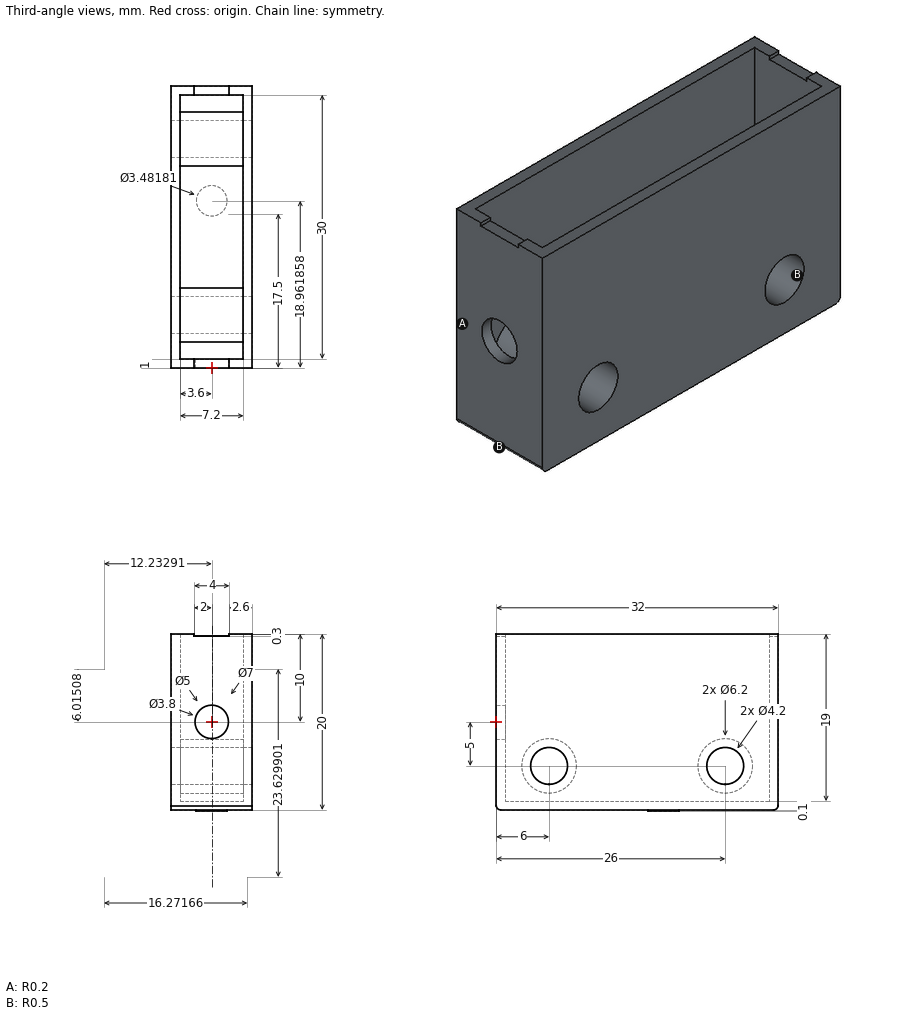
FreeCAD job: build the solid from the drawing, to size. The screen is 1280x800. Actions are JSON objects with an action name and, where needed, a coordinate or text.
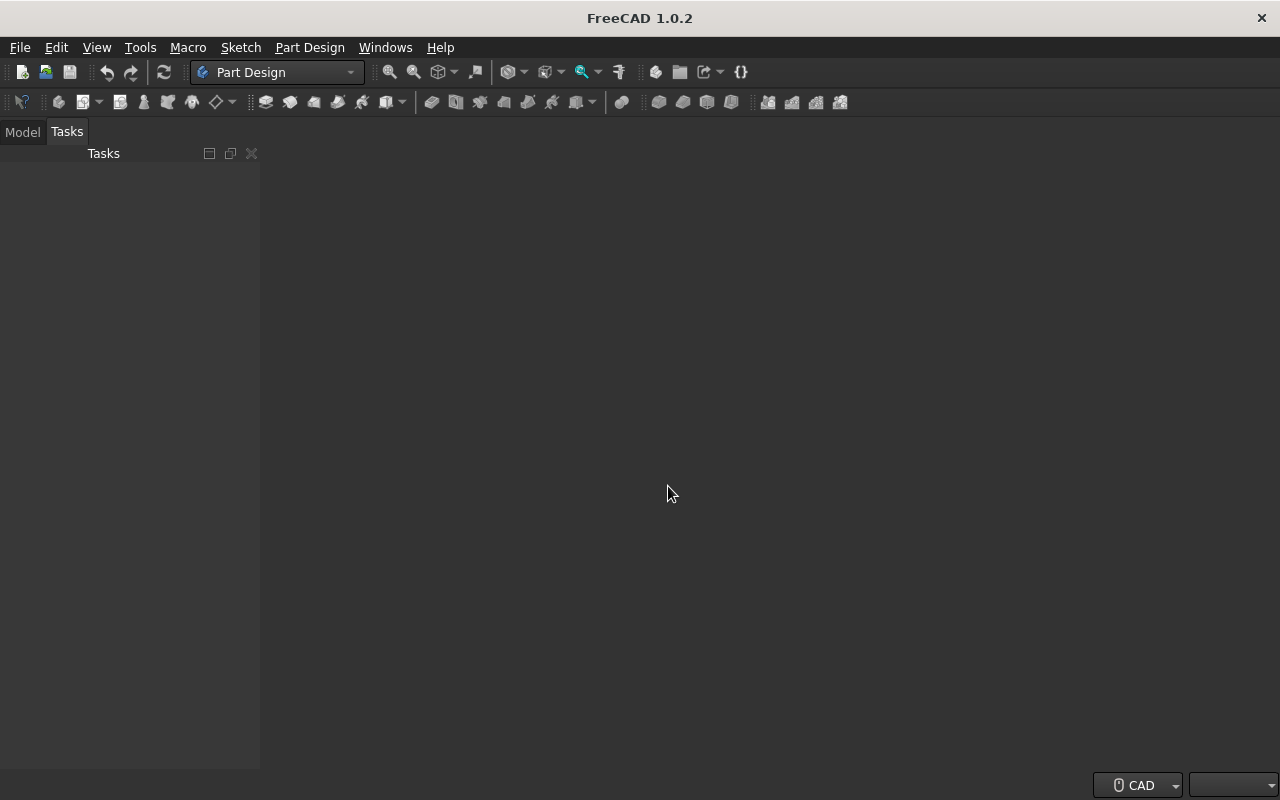
{"action": "left_click", "coordinate": [22, 72]}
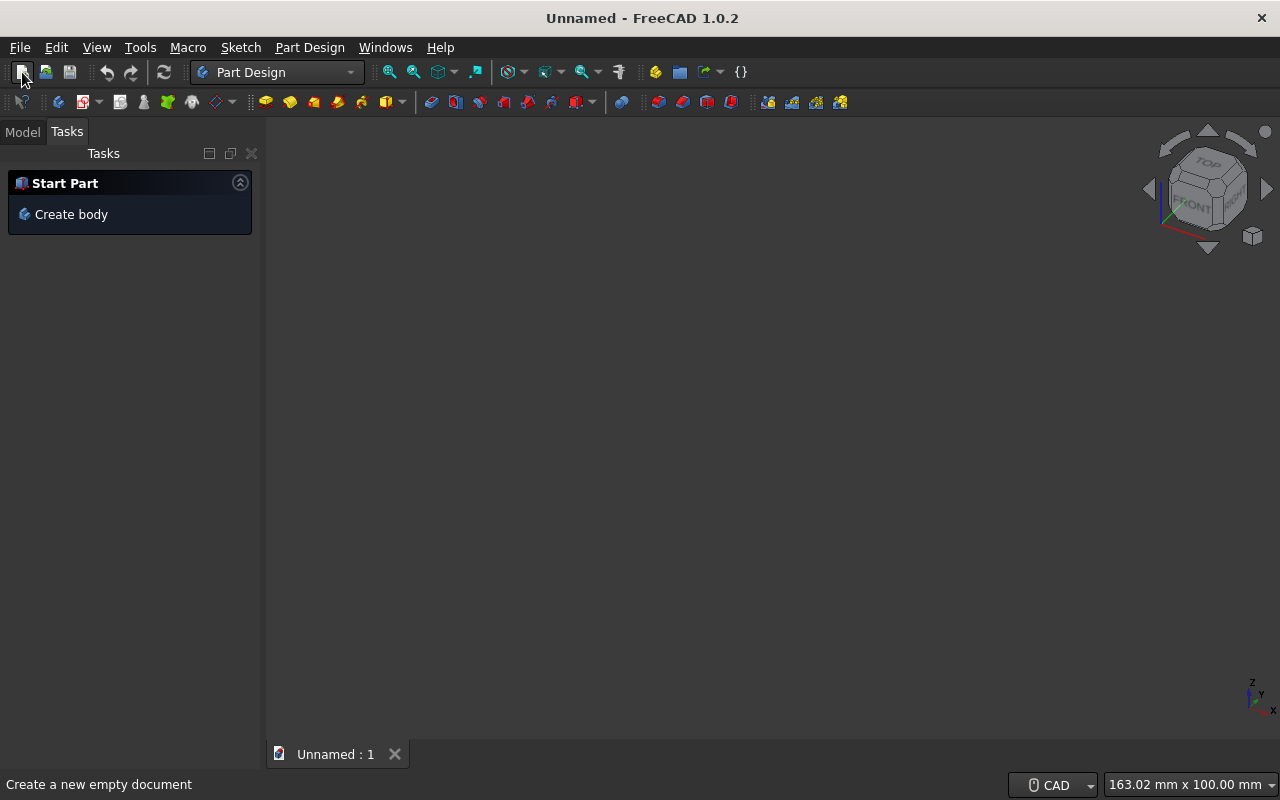
{"action": "left_click", "coordinate": [84, 102]}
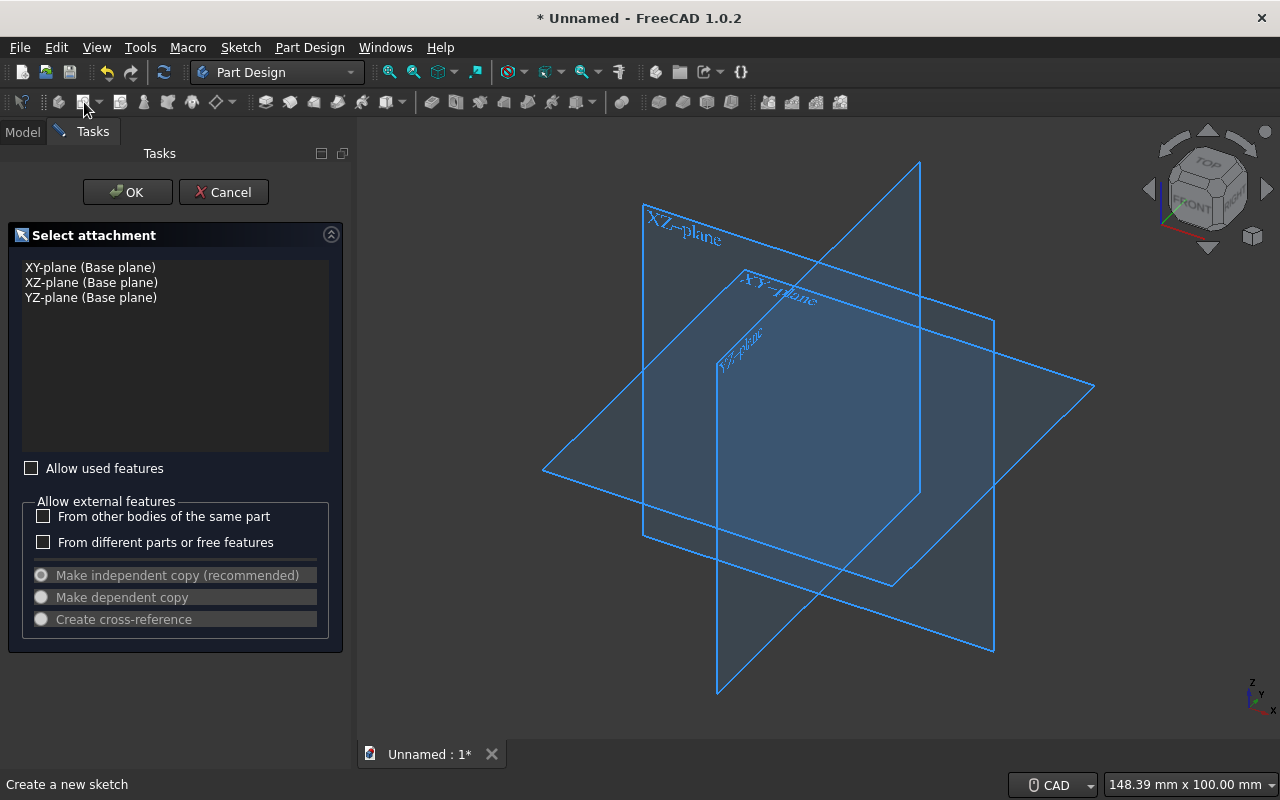
{"action": "left_click", "coordinate": [82, 282]}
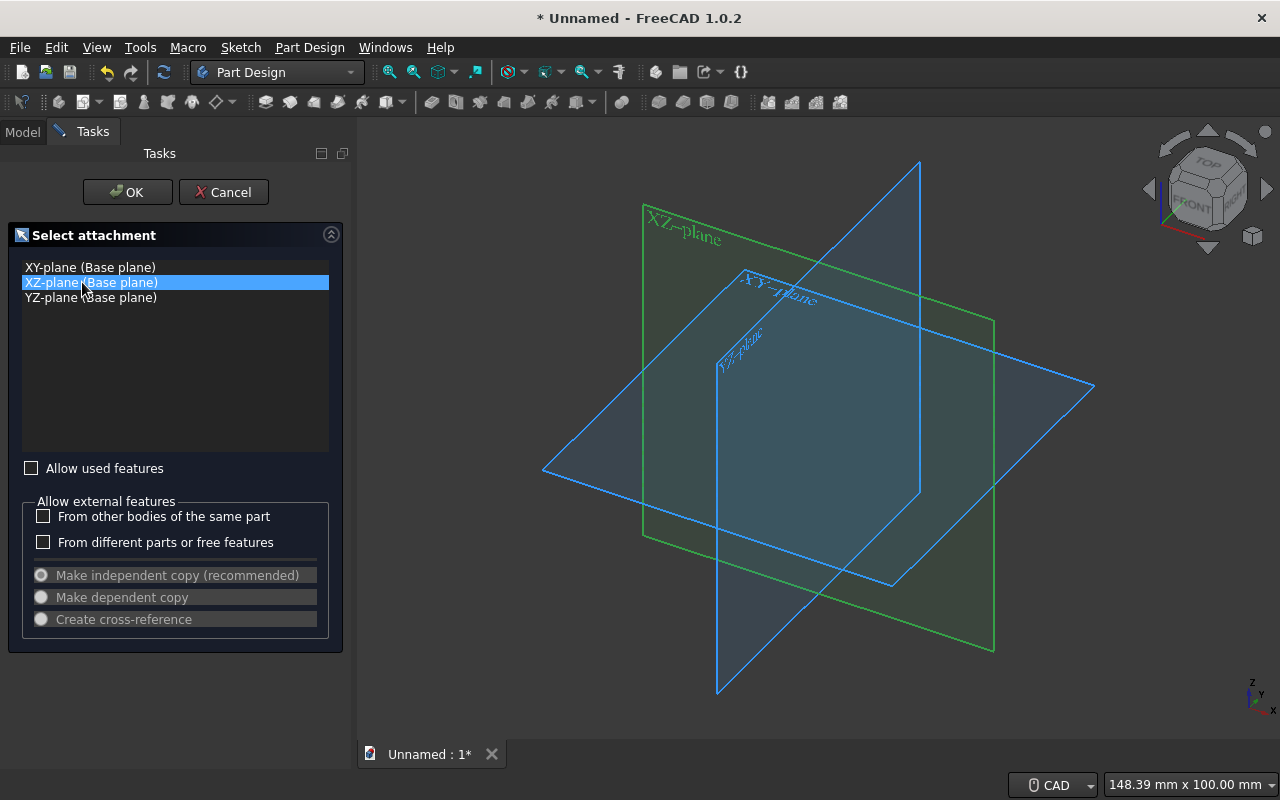
{"action": "left_click", "coordinate": [128, 192]}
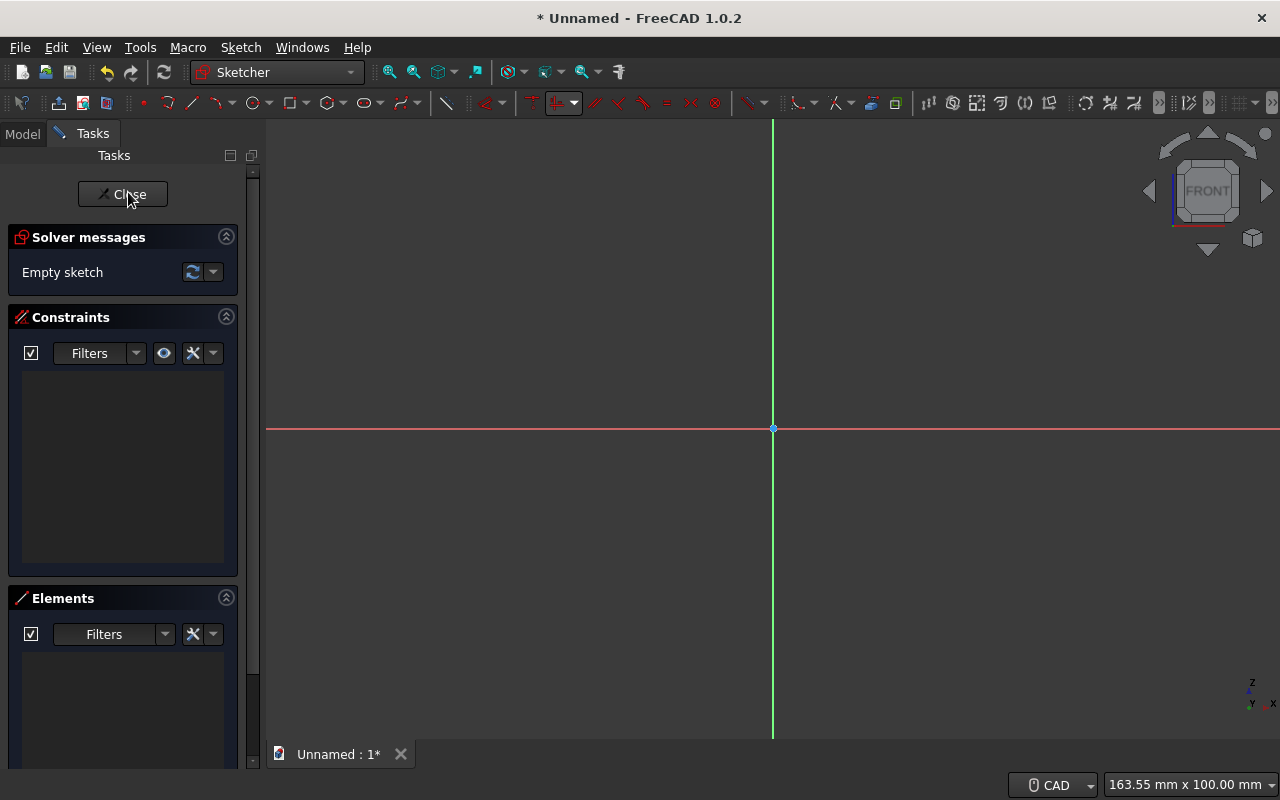
{"action": "scroll", "coordinate": [803, 429], "scroll_direction": "up", "scroll_amount": 6}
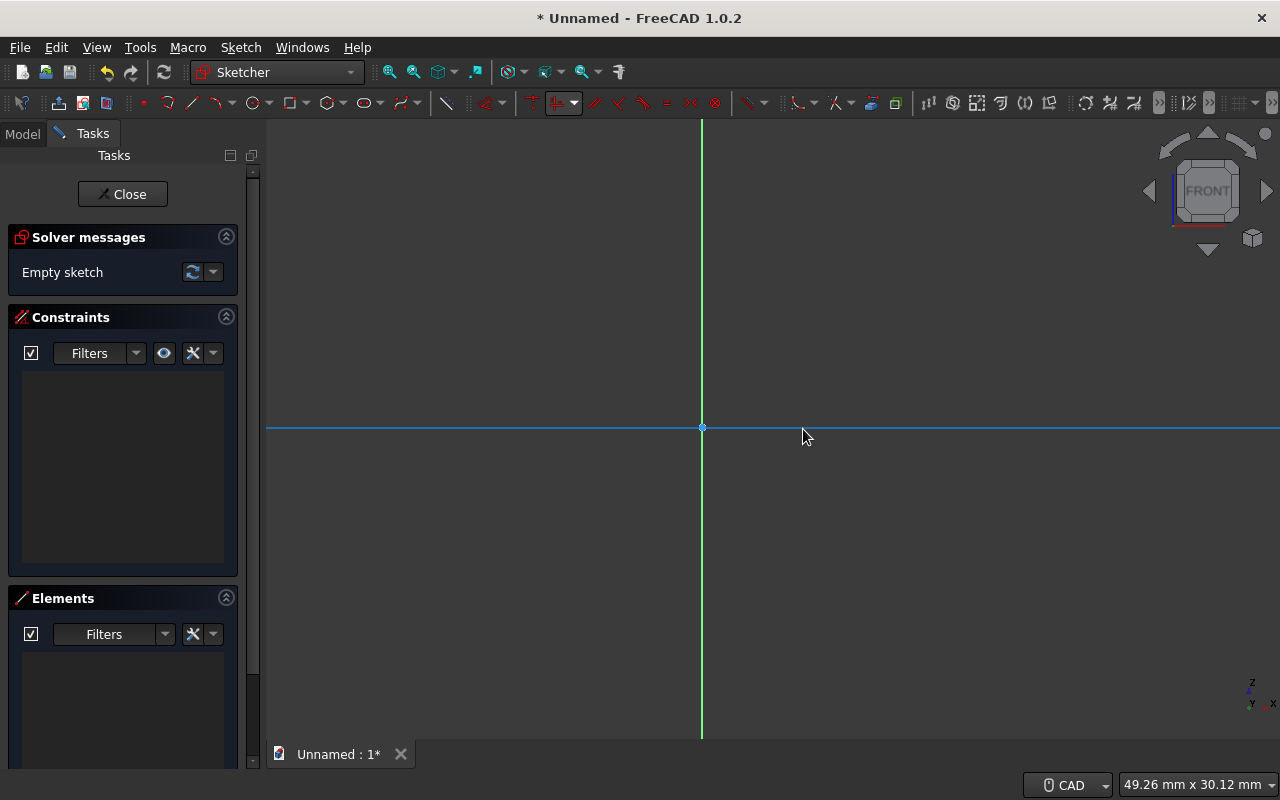
{"action": "left_click", "coordinate": [168, 104]}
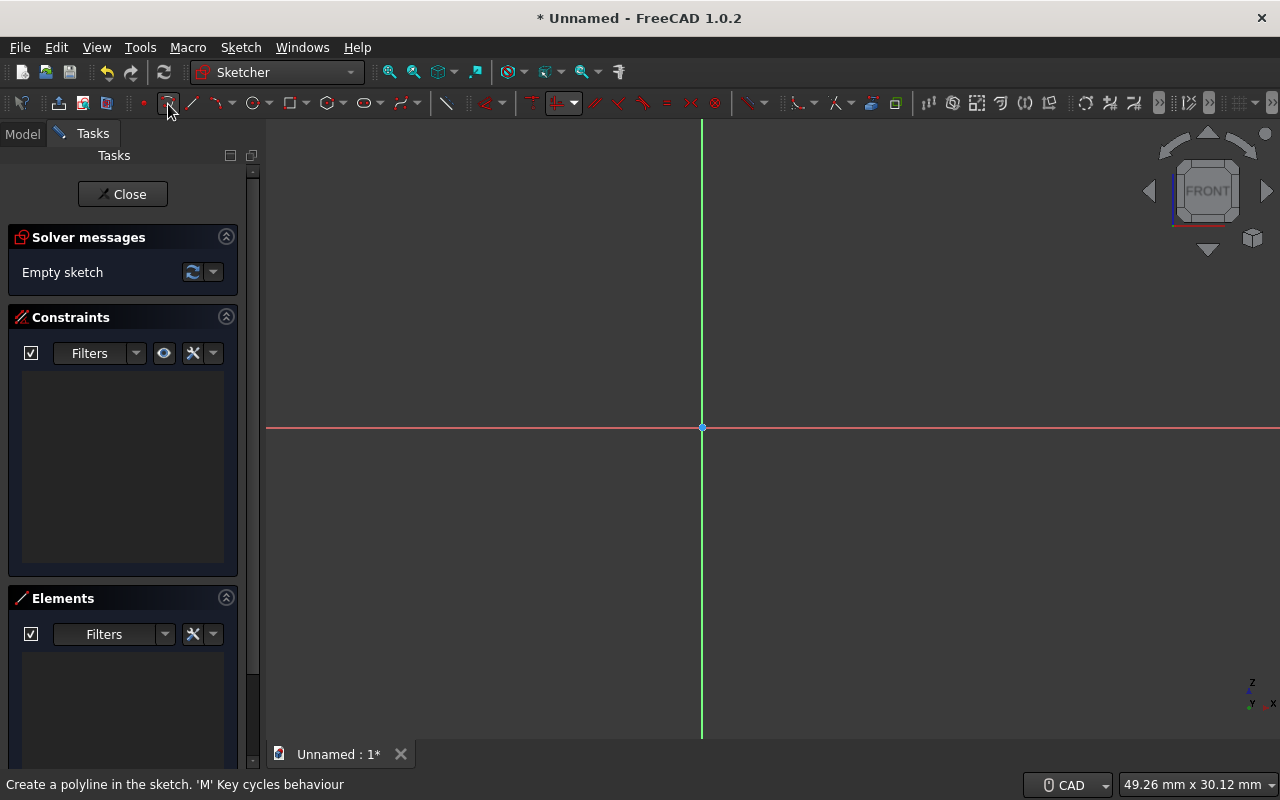
{"action": "left_click", "coordinate": [661, 228]}
{"action": "left_click", "coordinate": [743, 228]}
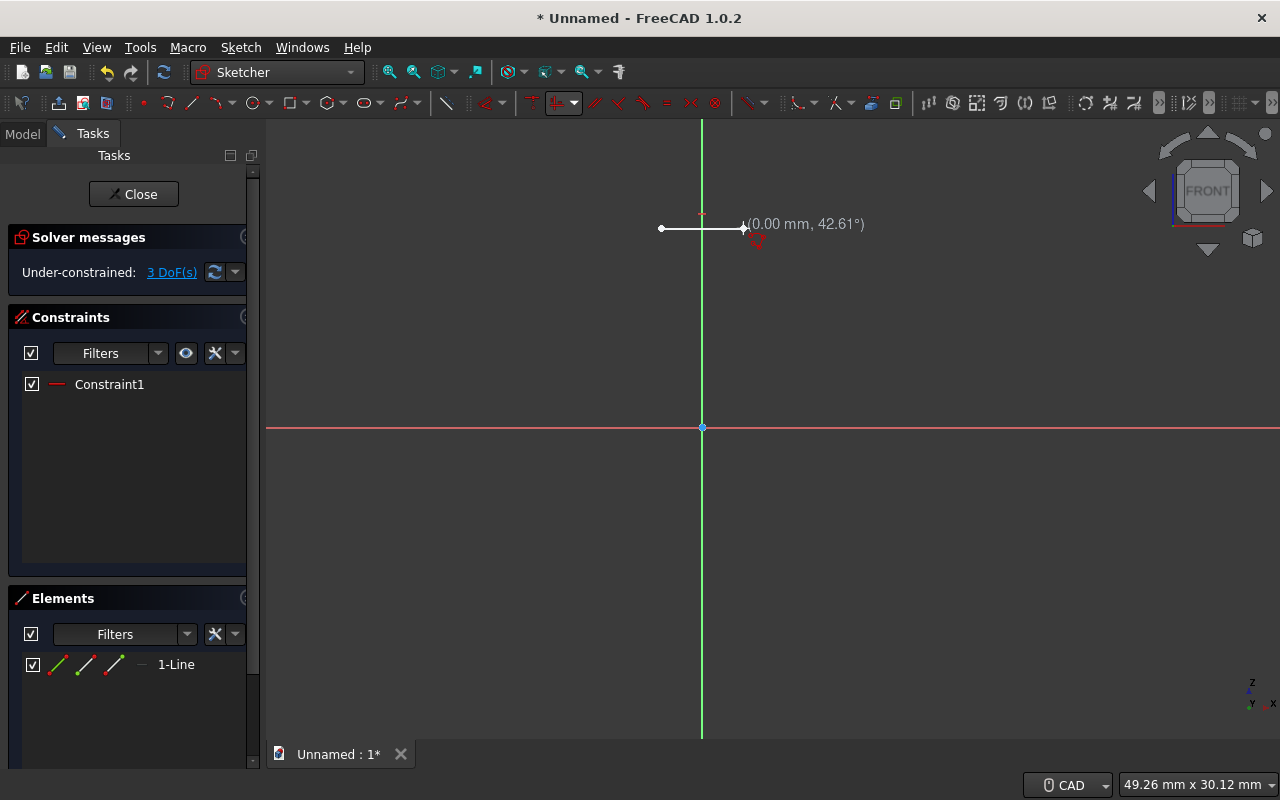
{"action": "scroll", "coordinate": [743, 222], "scroll_direction": "up", "scroll_amount": 5}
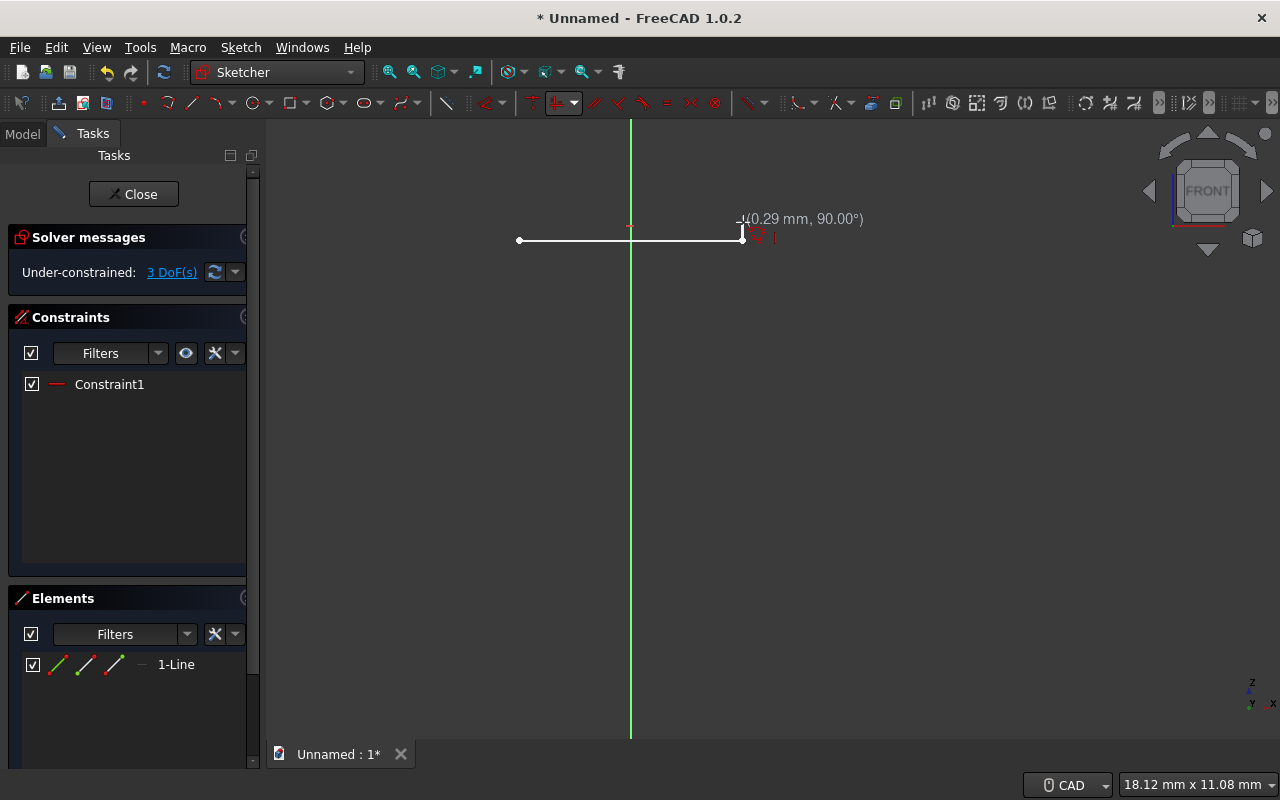
{"action": "left_click", "coordinate": [742, 222]}
{"action": "left_click", "coordinate": [889, 222]}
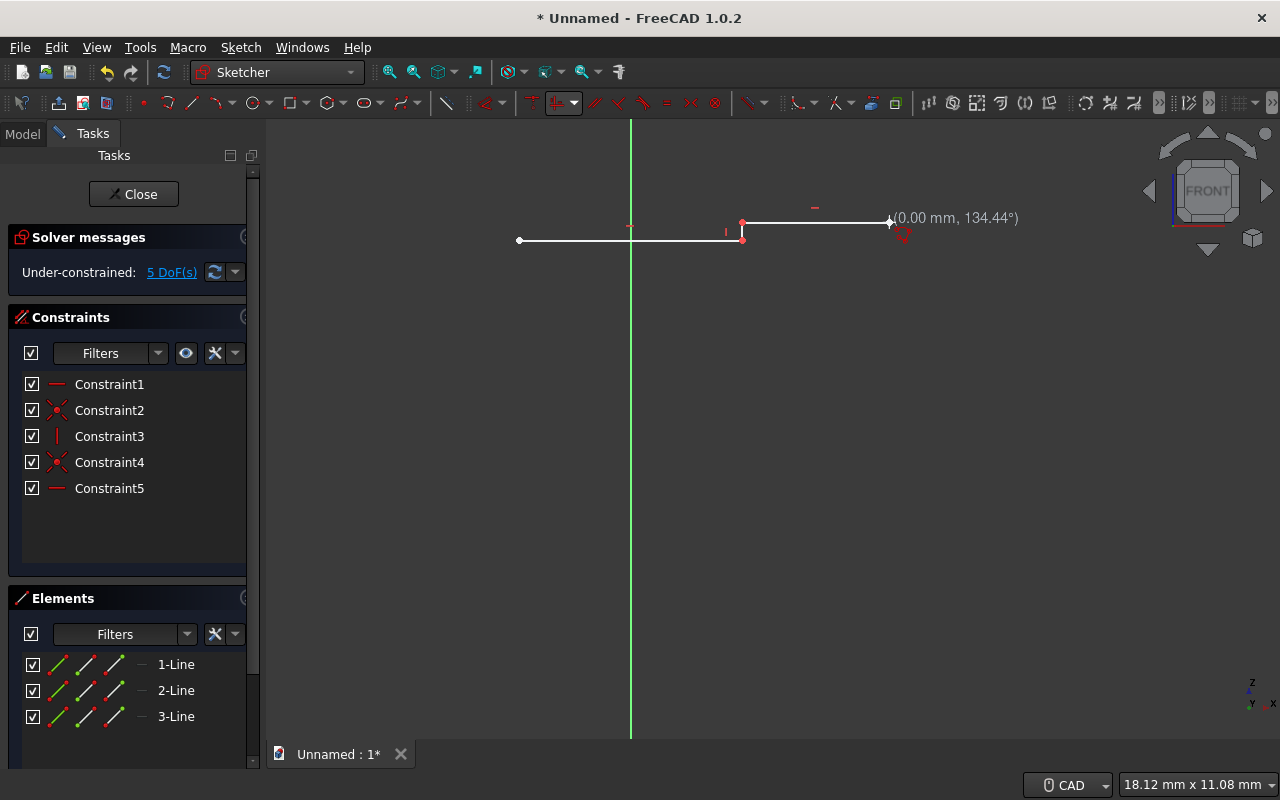
{"action": "scroll", "coordinate": [747, 224], "scroll_direction": "down", "scroll_amount": 5}